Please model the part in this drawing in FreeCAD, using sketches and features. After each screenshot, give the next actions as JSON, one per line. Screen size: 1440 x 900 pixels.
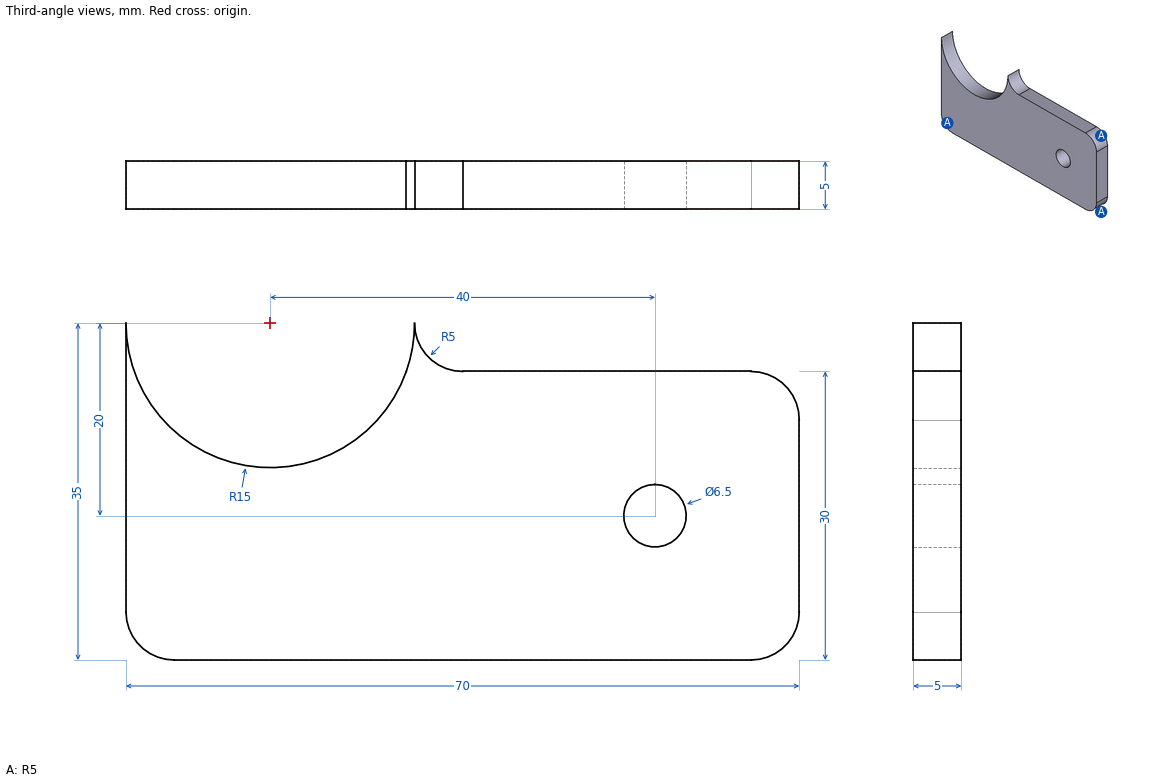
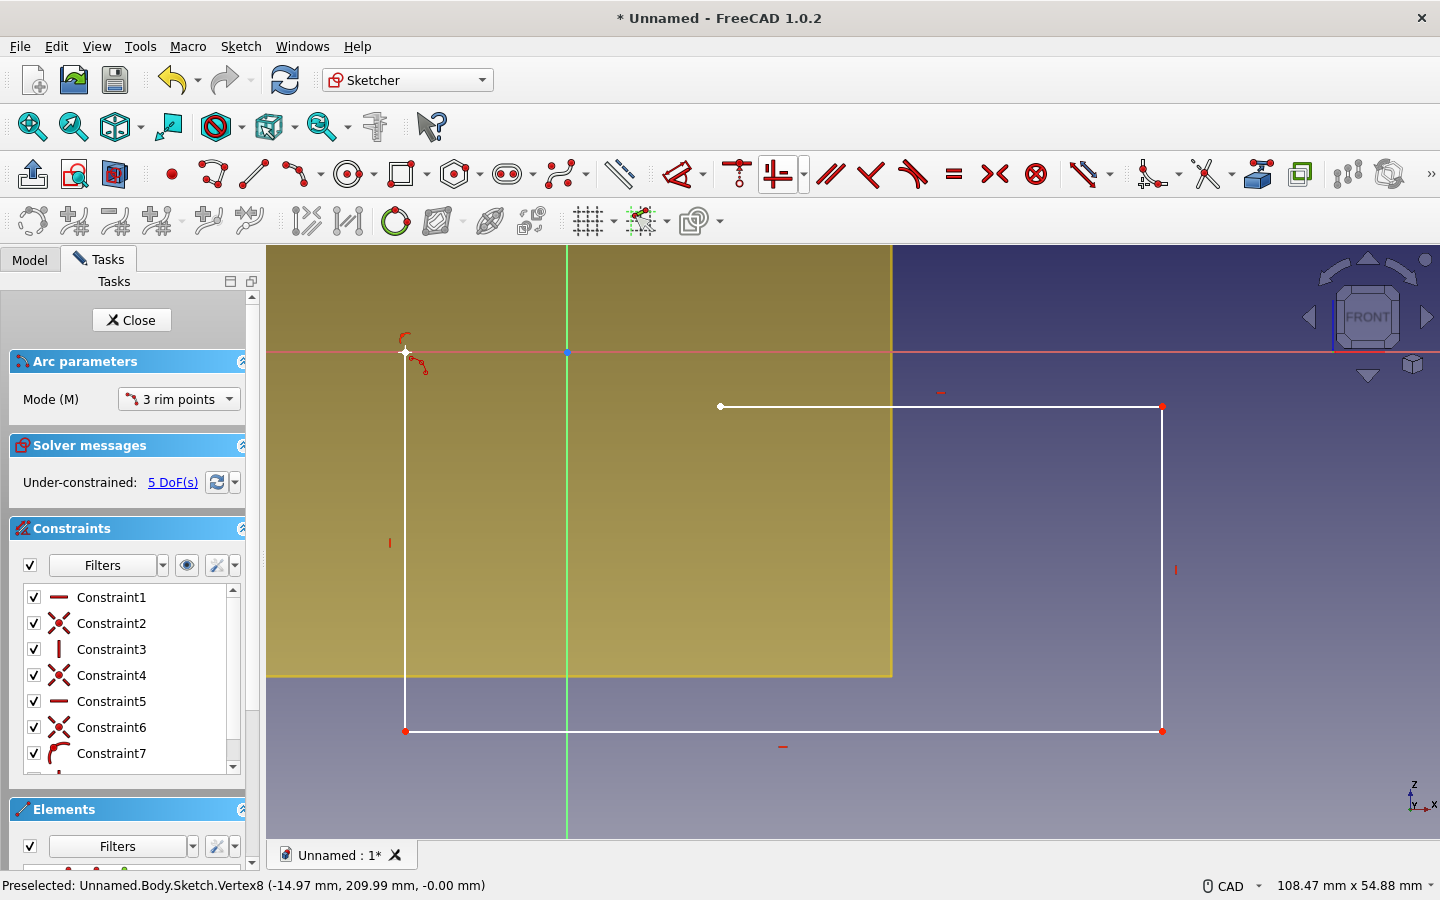
{"action": "left_click", "coordinate": [405, 352]}
{"action": "left_click", "coordinate": [720, 407]}
{"action": "left_click", "coordinate": [540, 512]}
{"action": "key", "text": "Escape"}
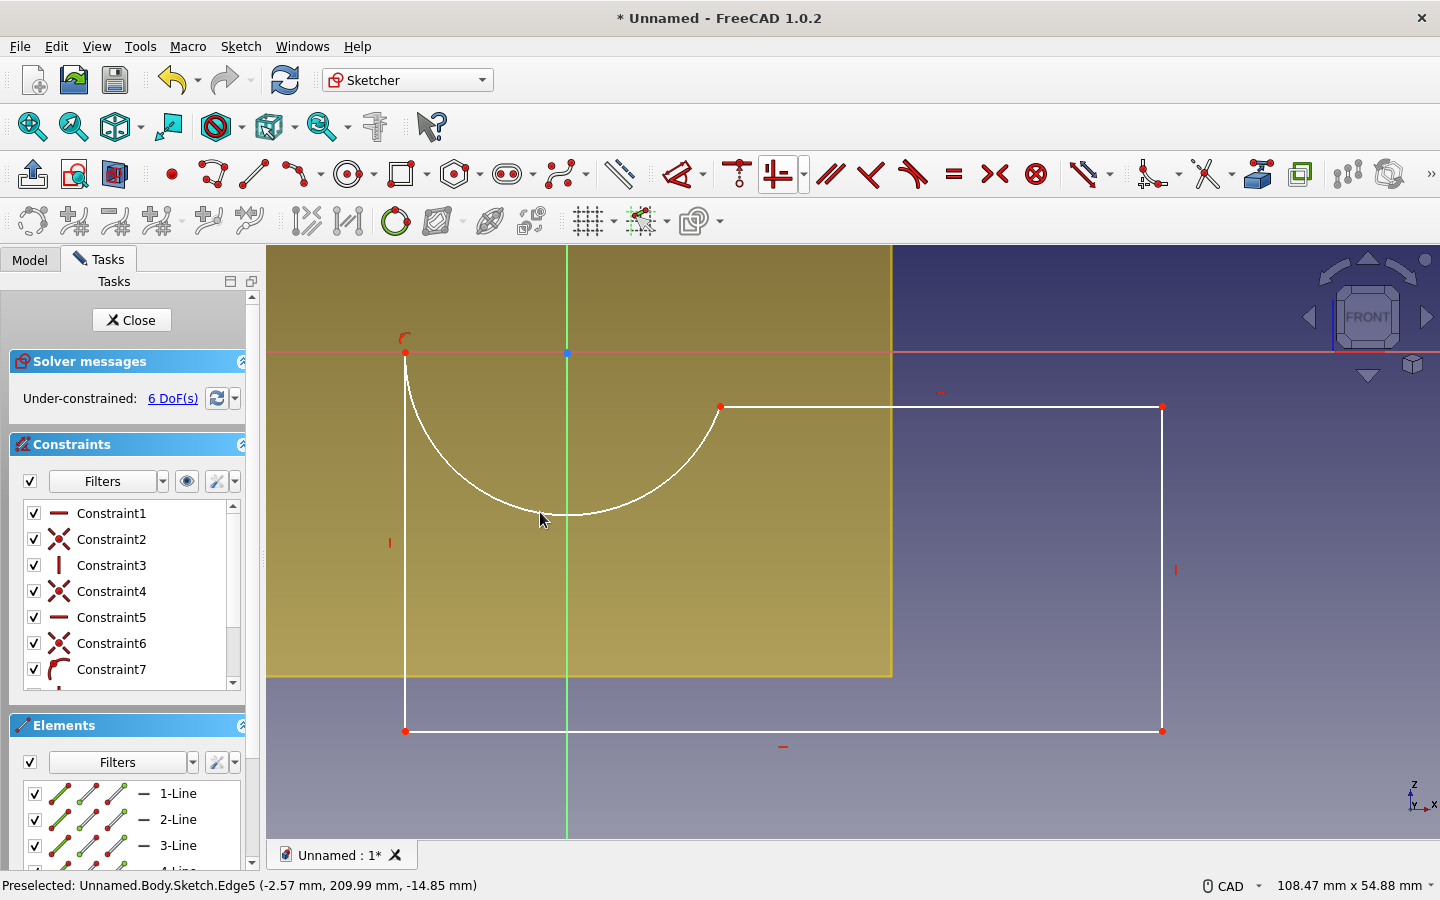
{"action": "left_click", "coordinate": [405, 618]}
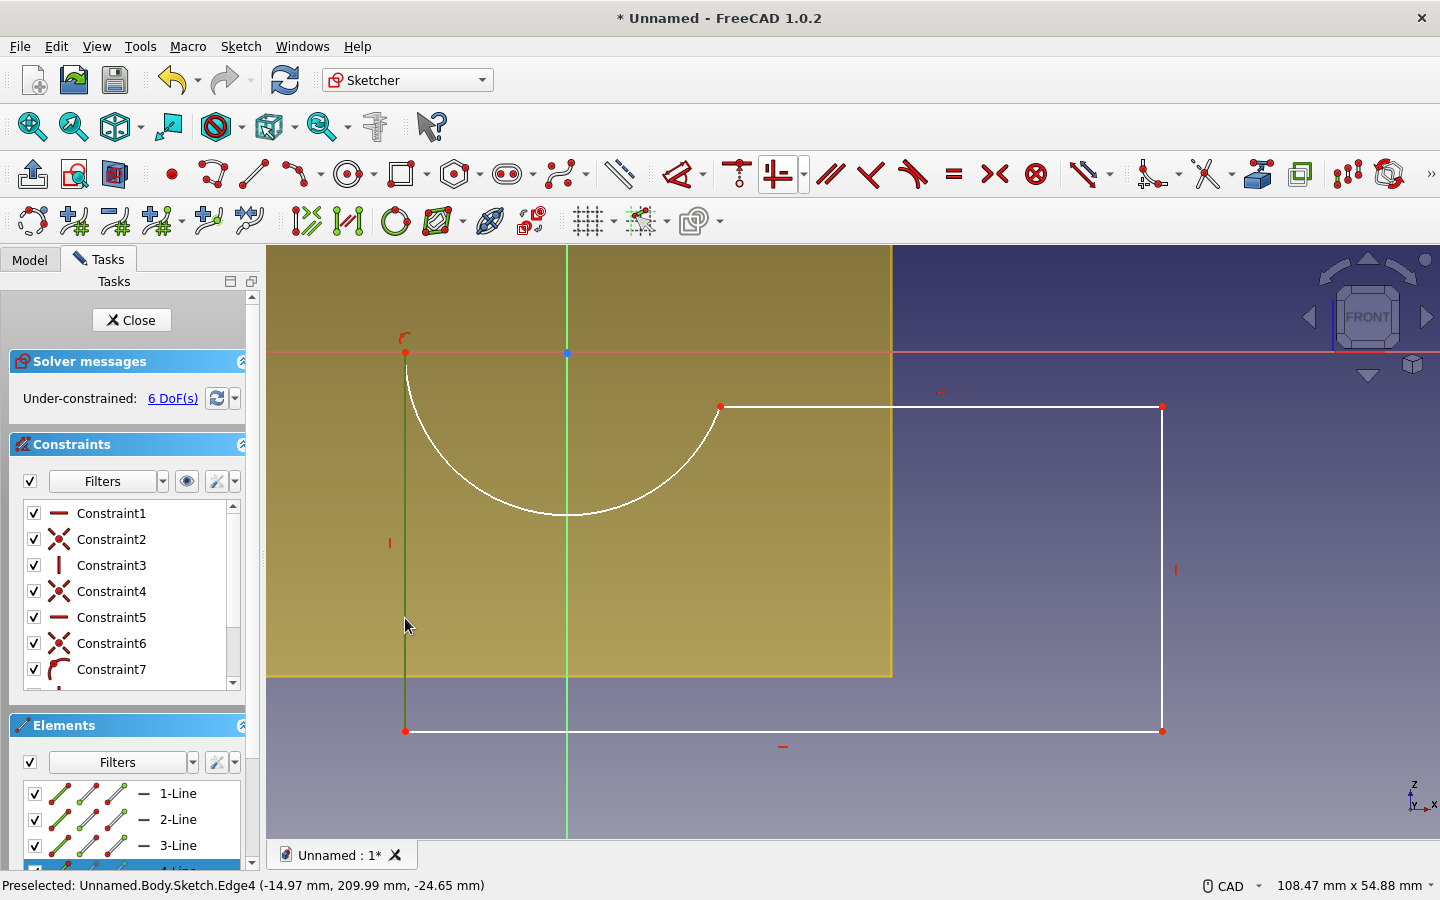
{"action": "left_click", "coordinate": [458, 474]}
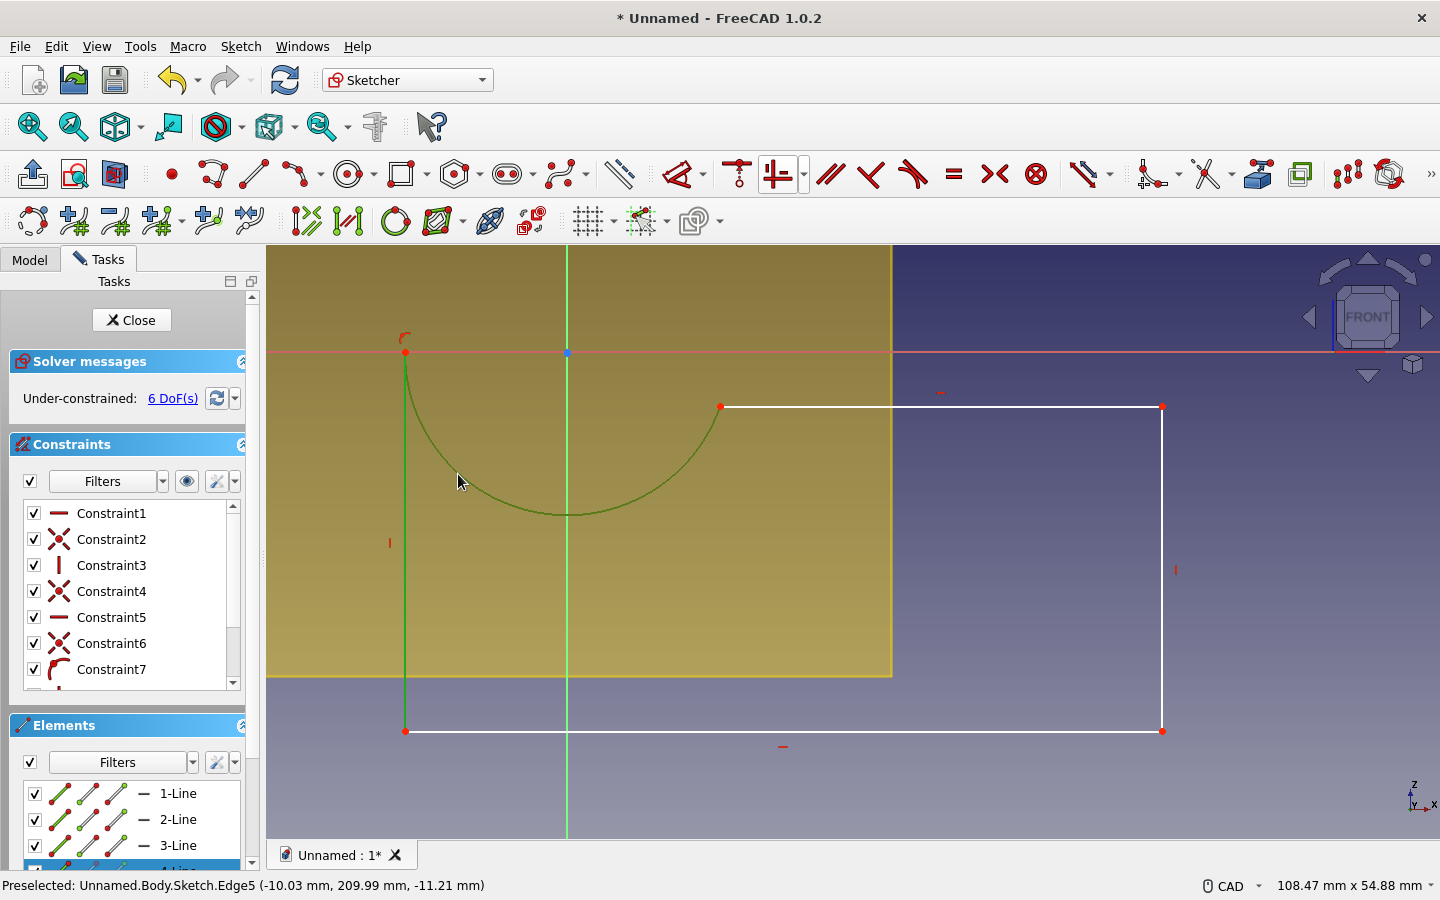
{"action": "left_click", "coordinate": [913, 174]}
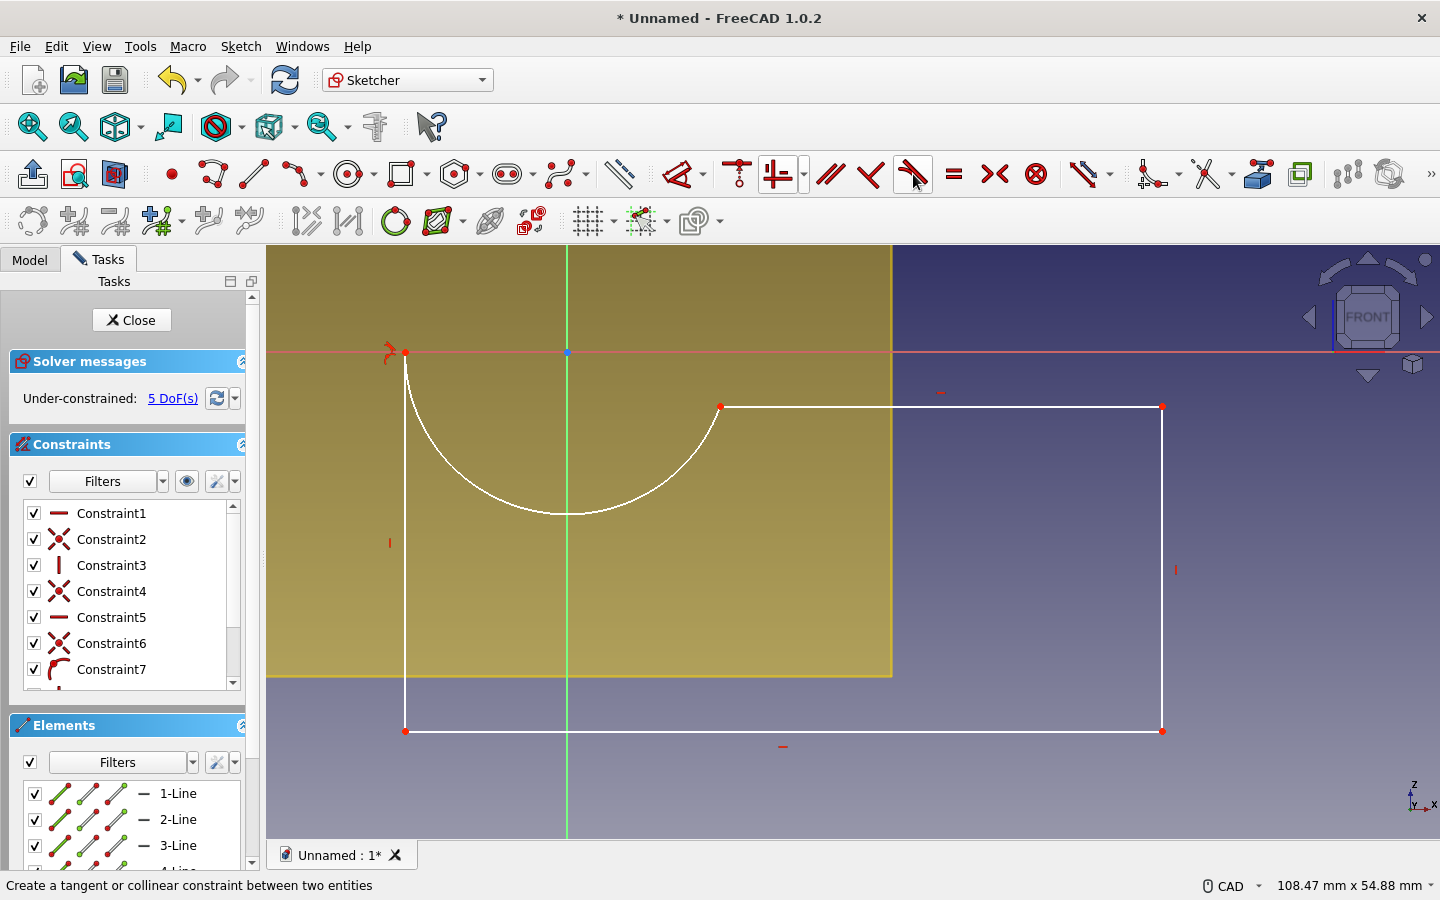
{"action": "left_click", "coordinate": [567, 352]}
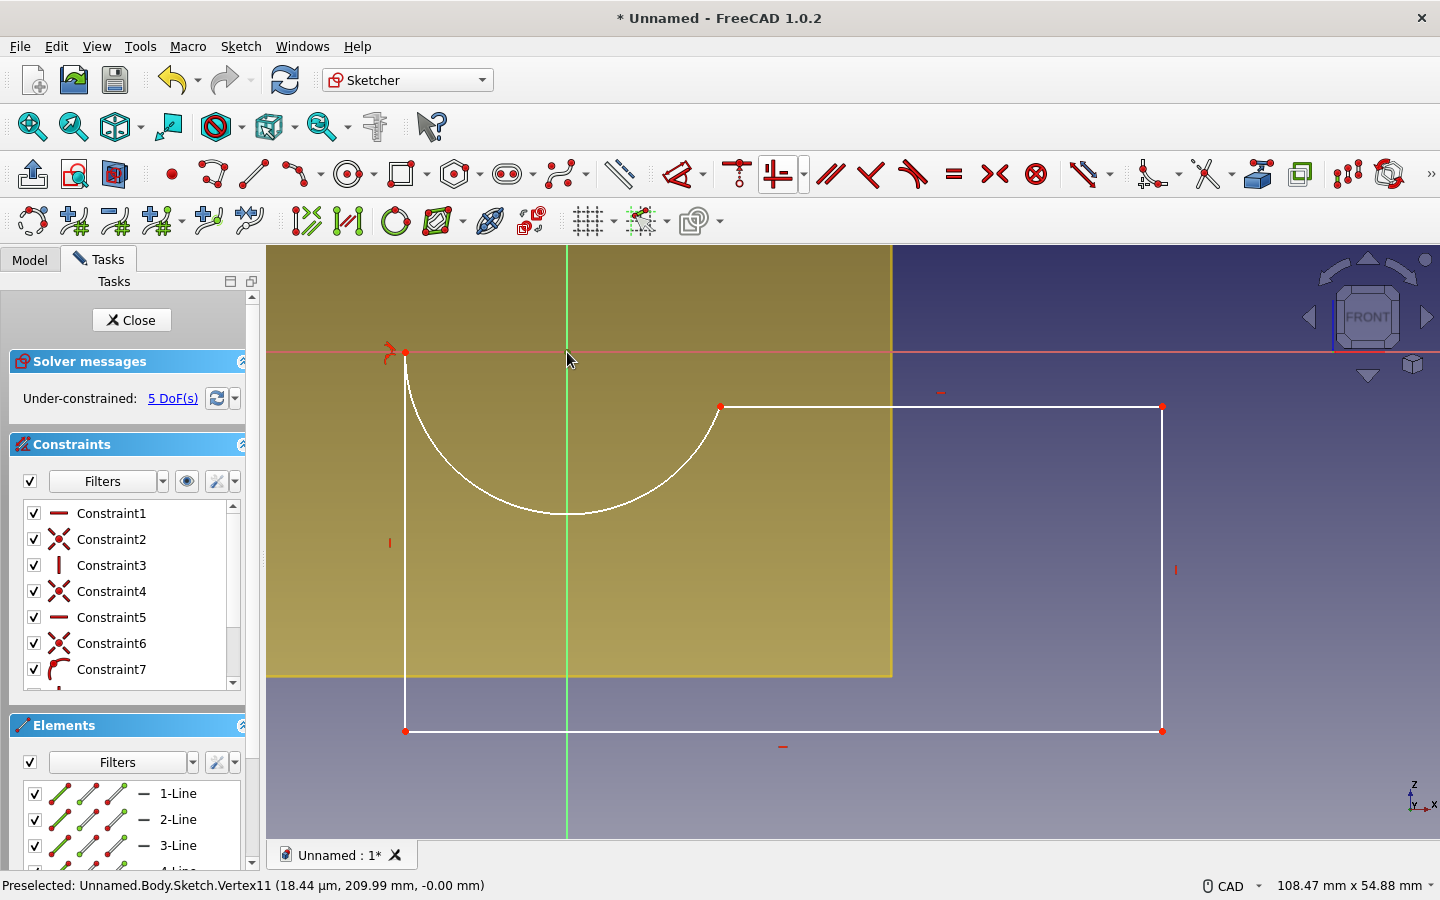
{"action": "left_click", "coordinate": [567, 773]}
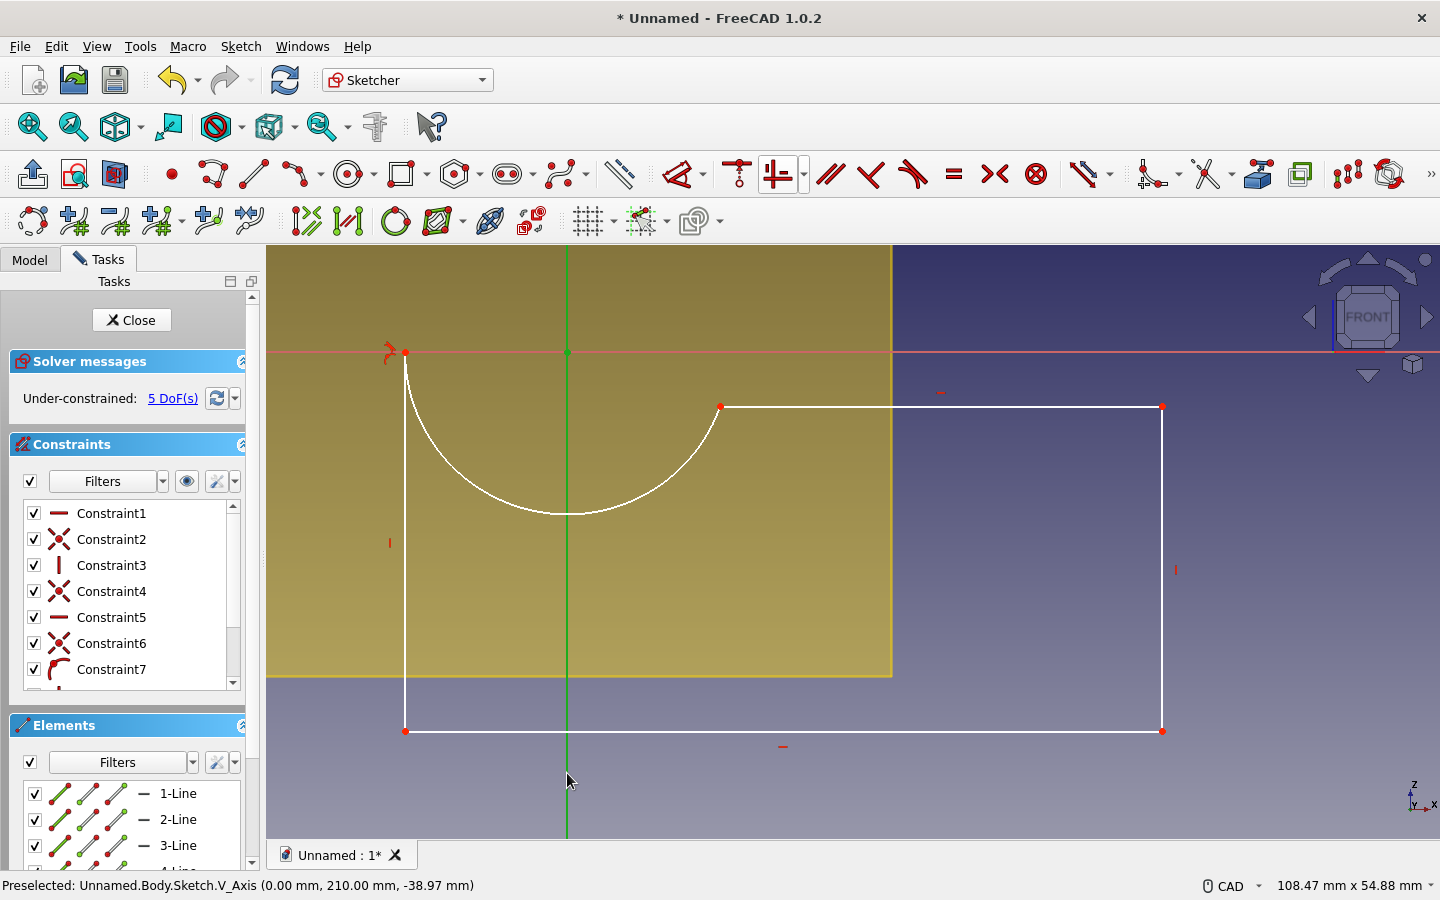
{"action": "left_click", "coordinate": [737, 174]}